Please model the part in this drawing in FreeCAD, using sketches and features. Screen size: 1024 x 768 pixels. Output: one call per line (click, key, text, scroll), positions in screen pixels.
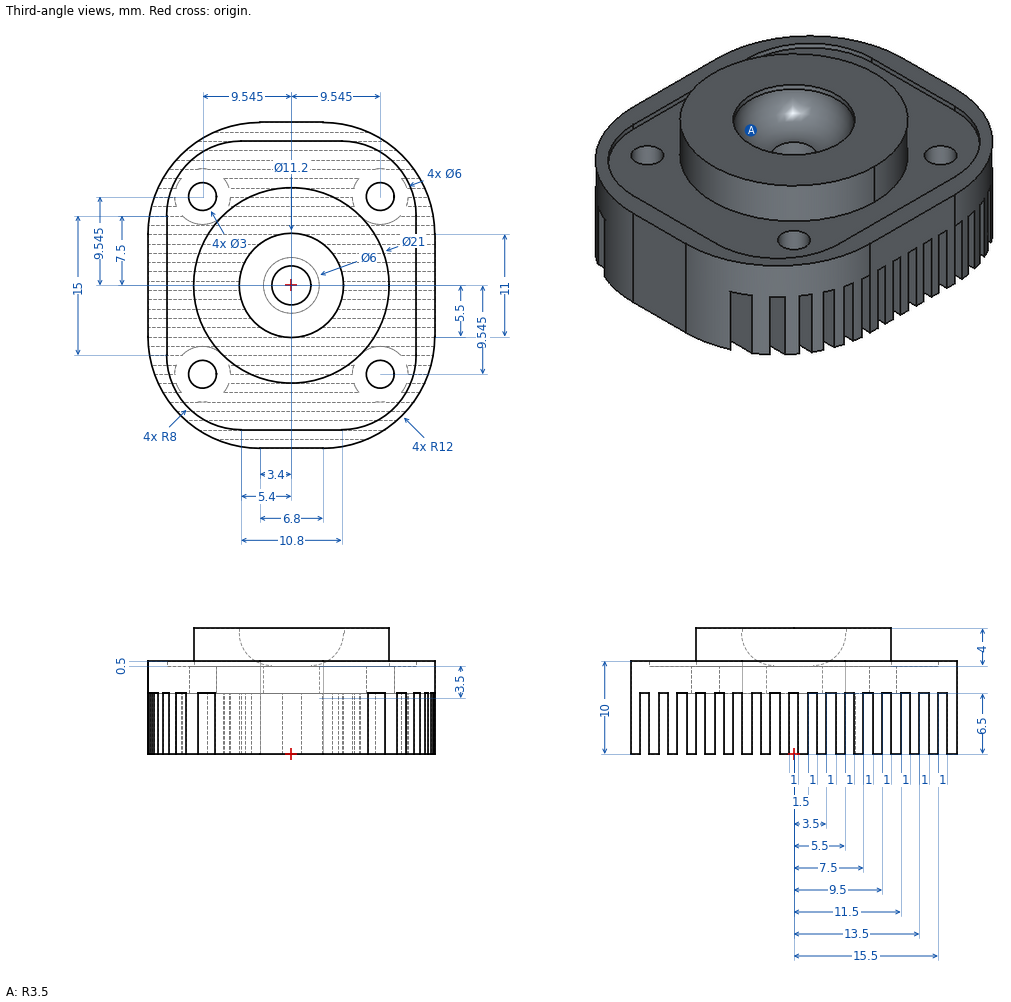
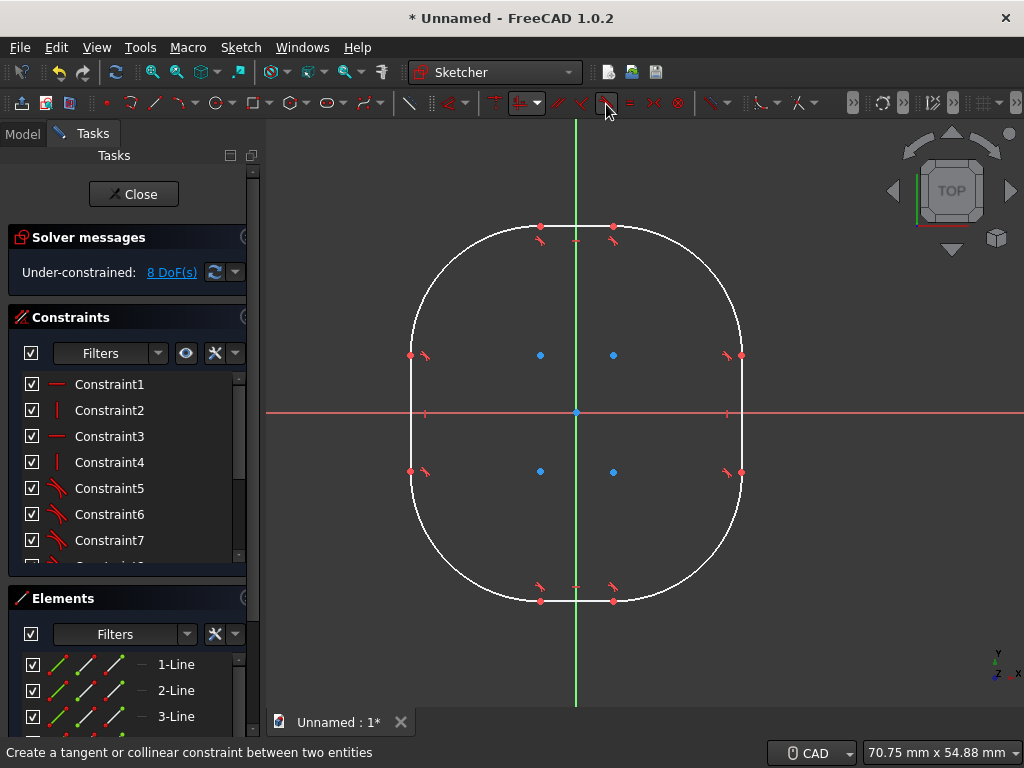
click(672, 587)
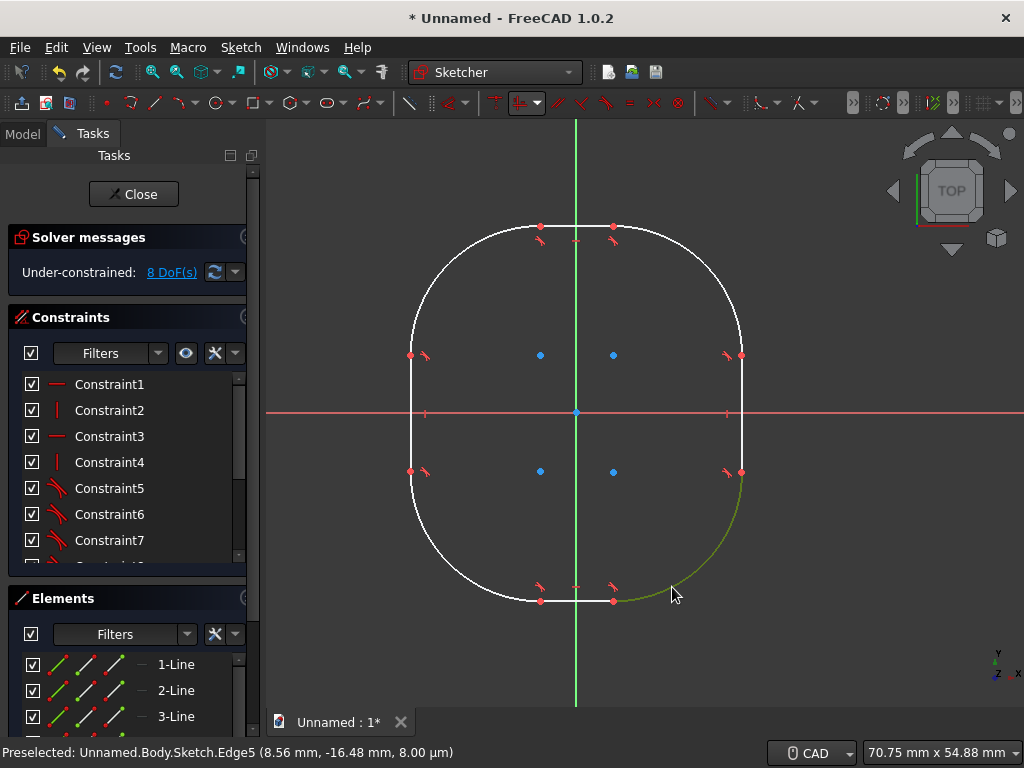
click(728, 296)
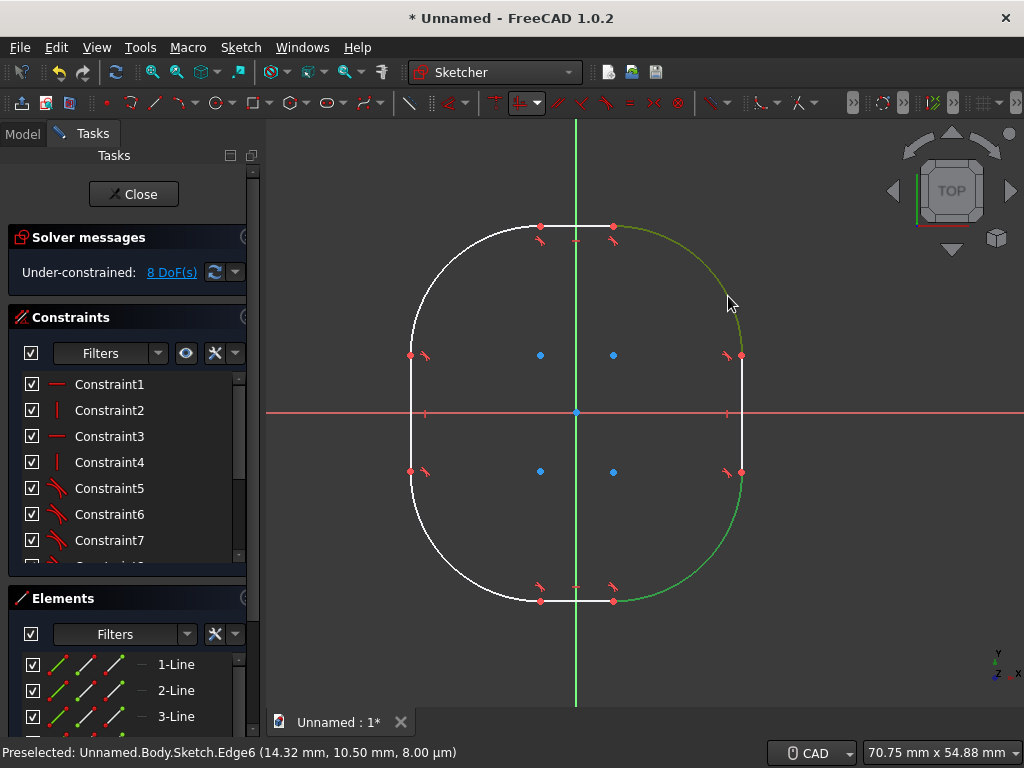
click(481, 240)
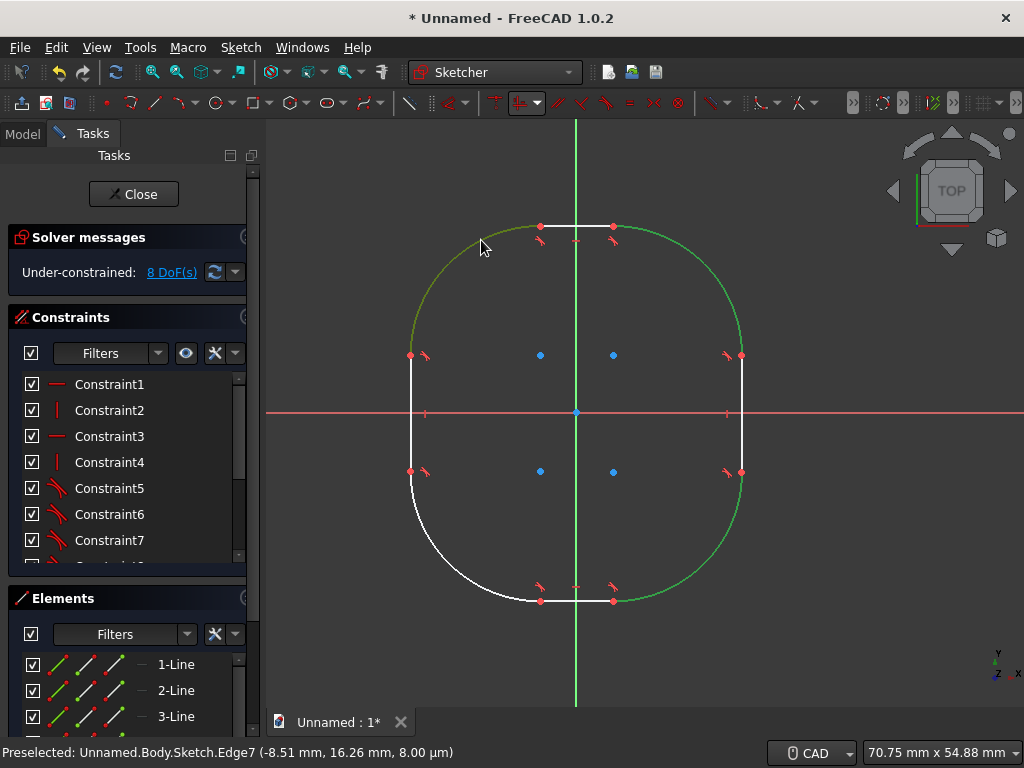
click(425, 530)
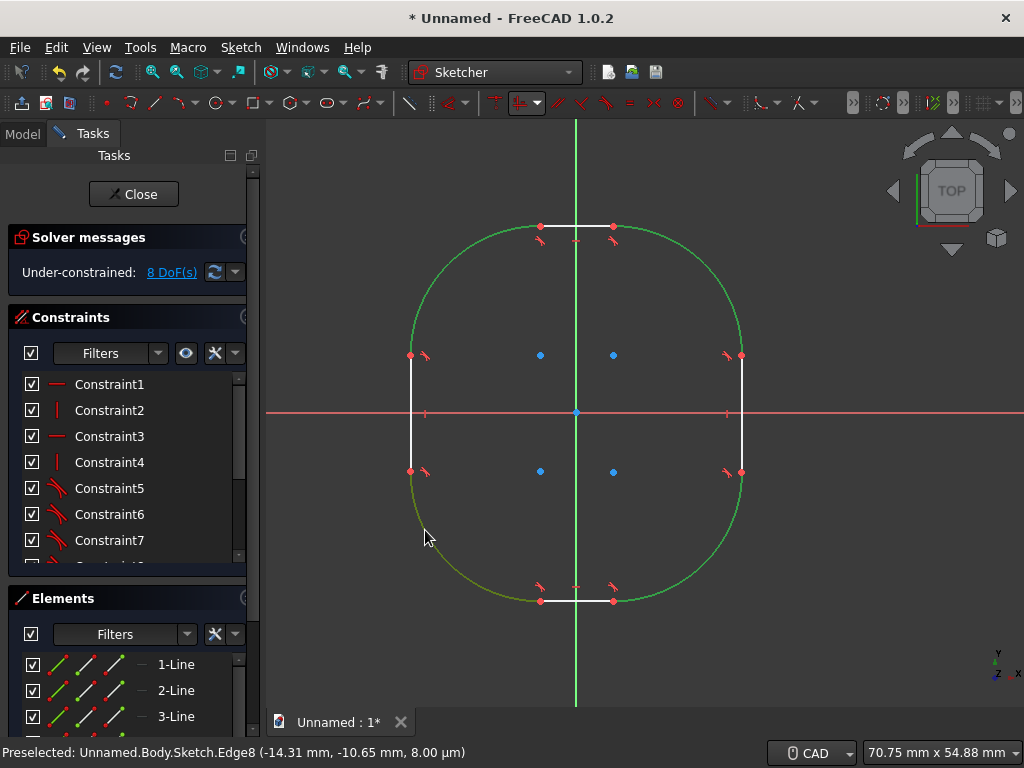
key(e)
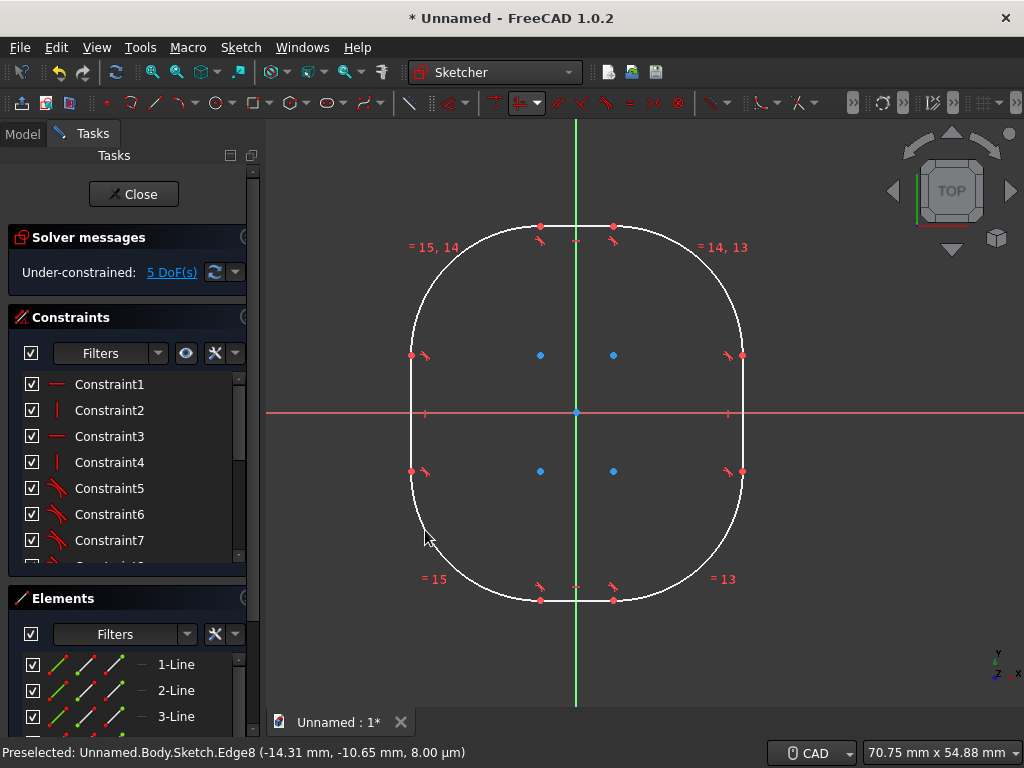
click(672, 587)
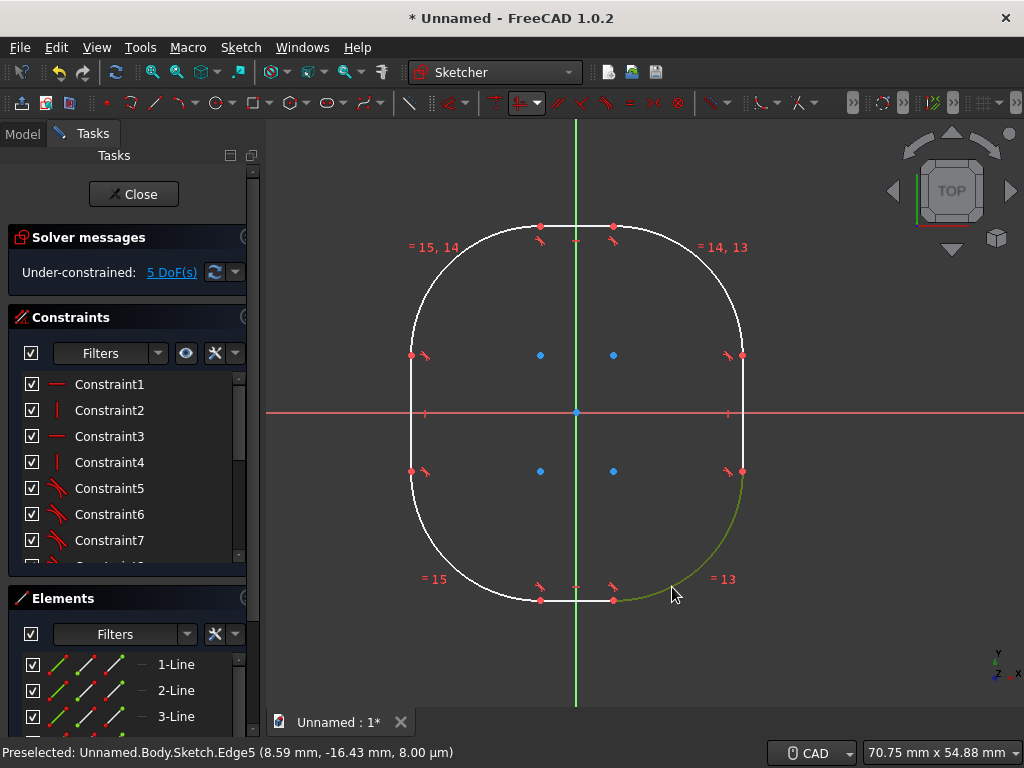
click(468, 104)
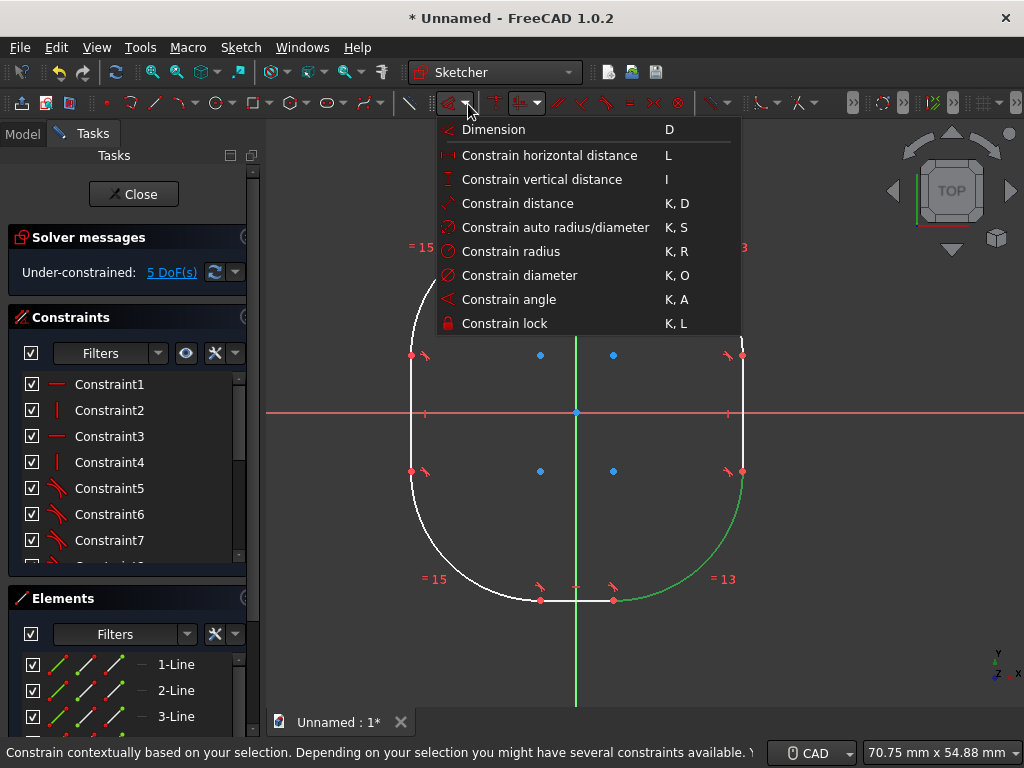
click(589, 251)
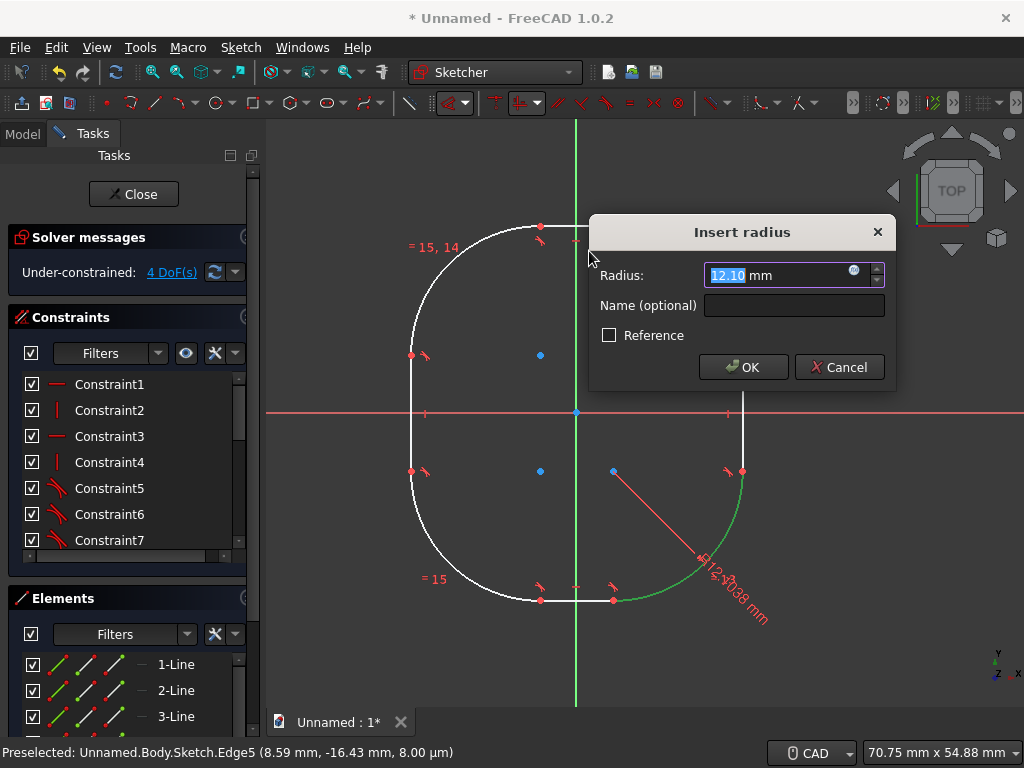
text(12)
key(Return)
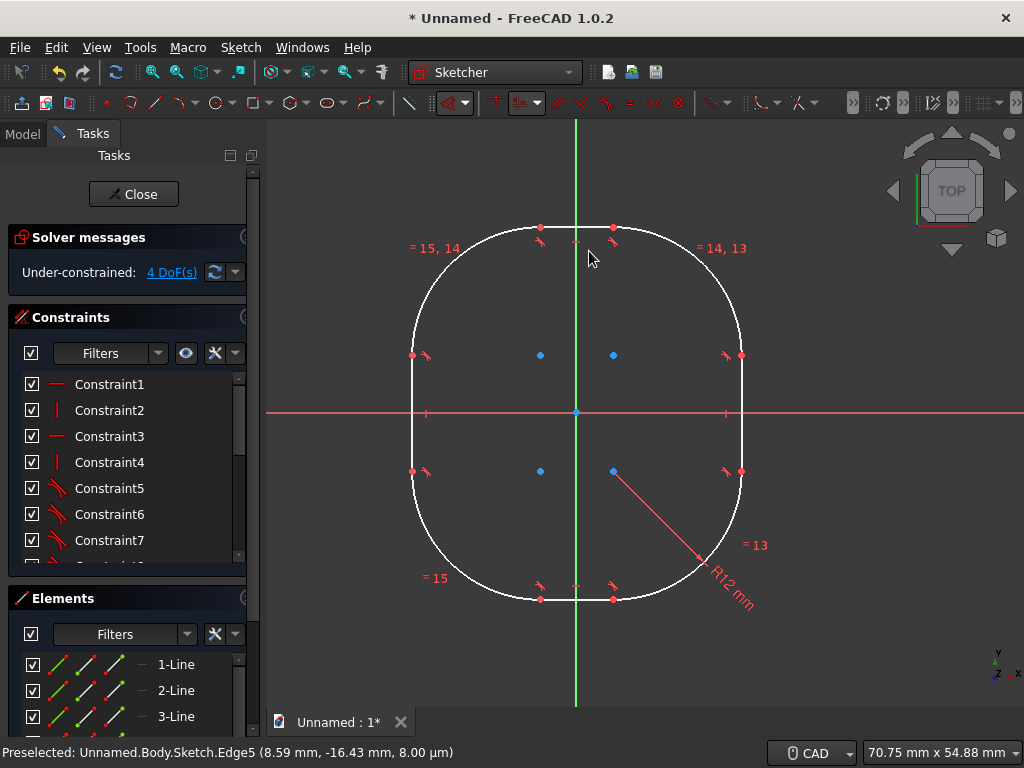
click(742, 437)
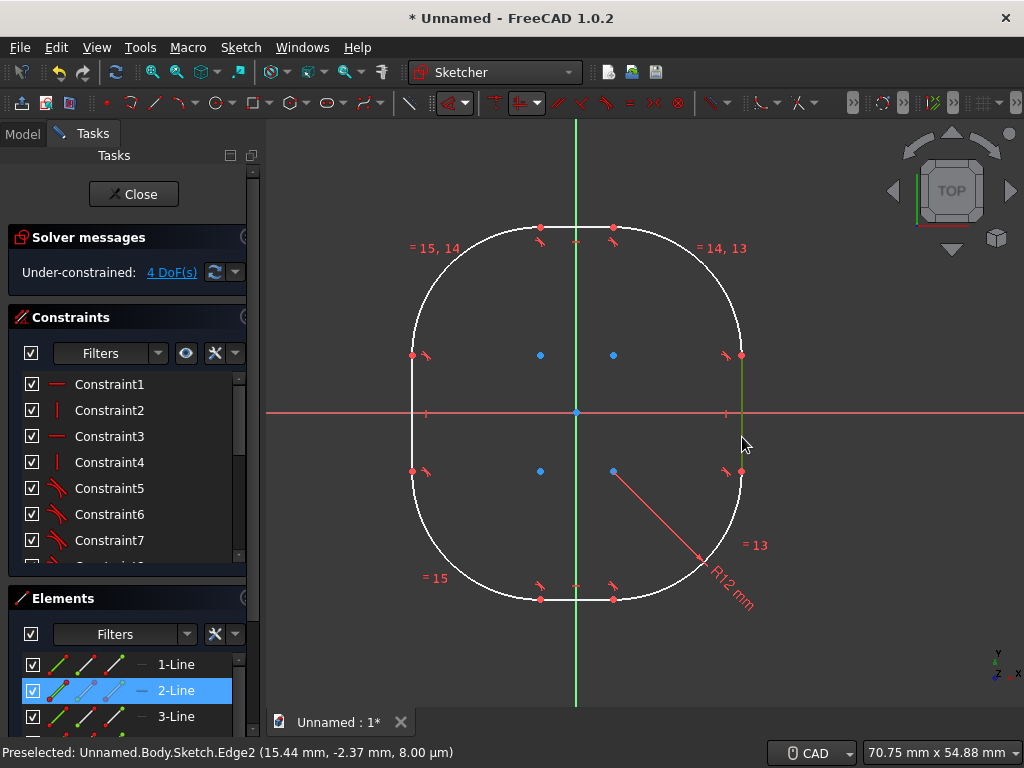
key(i)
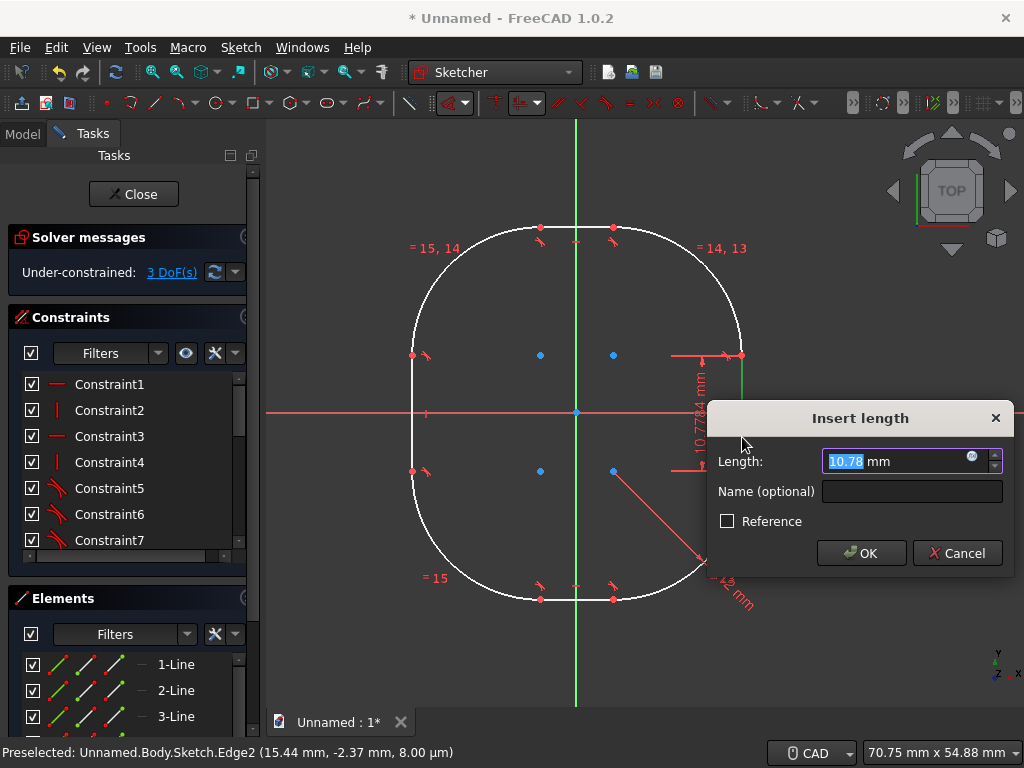
text(11)
key(Return)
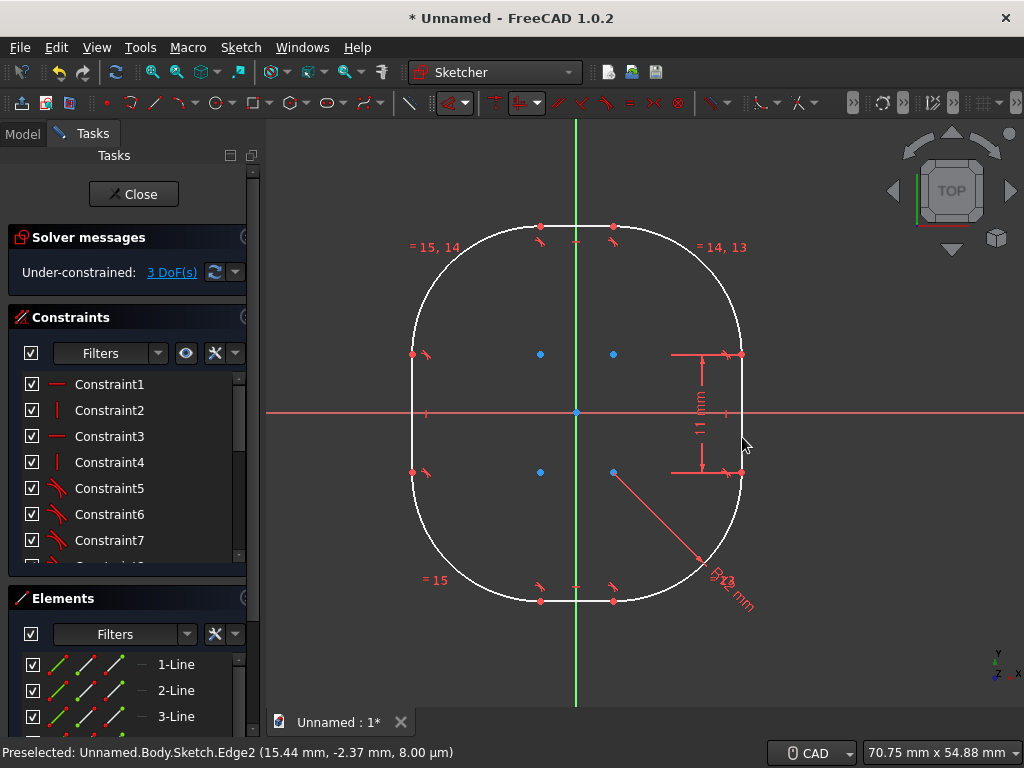
click(562, 601)